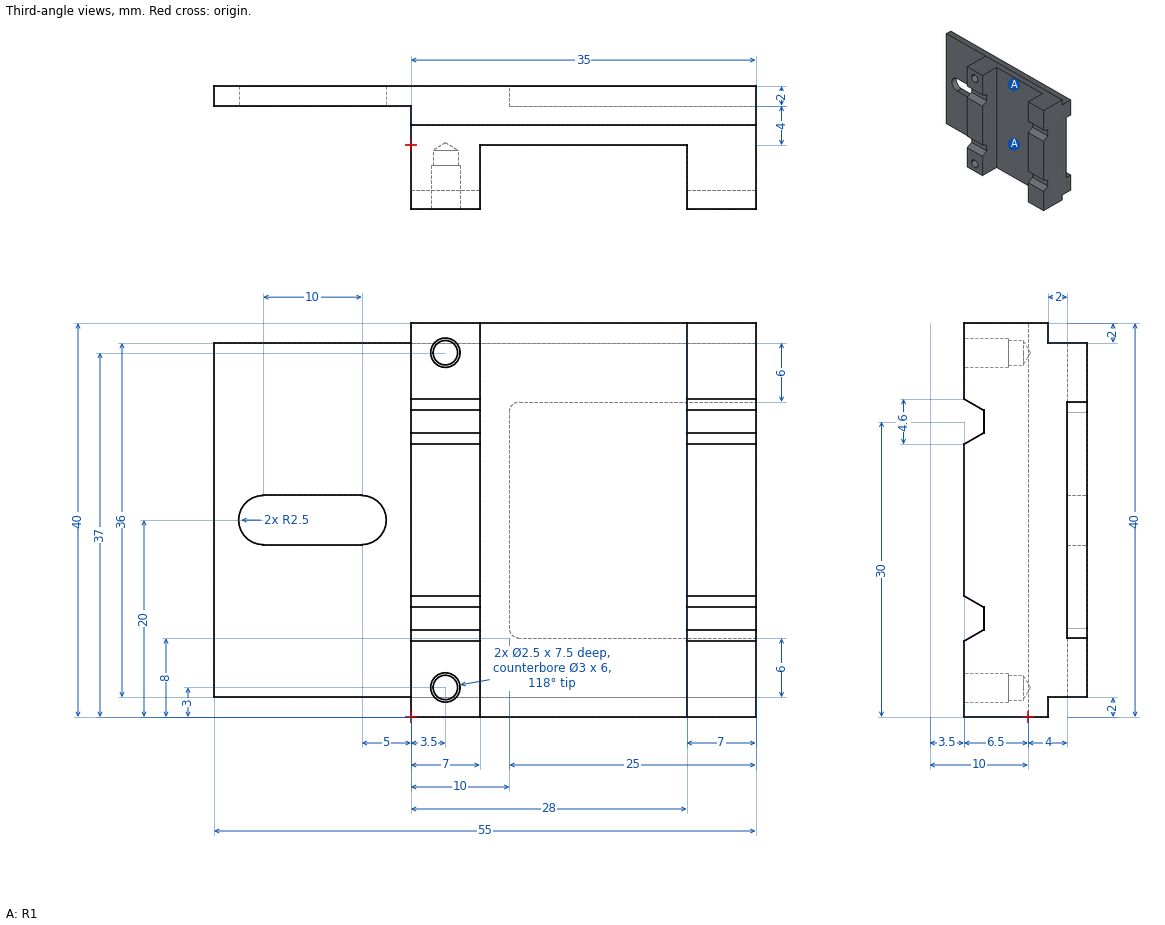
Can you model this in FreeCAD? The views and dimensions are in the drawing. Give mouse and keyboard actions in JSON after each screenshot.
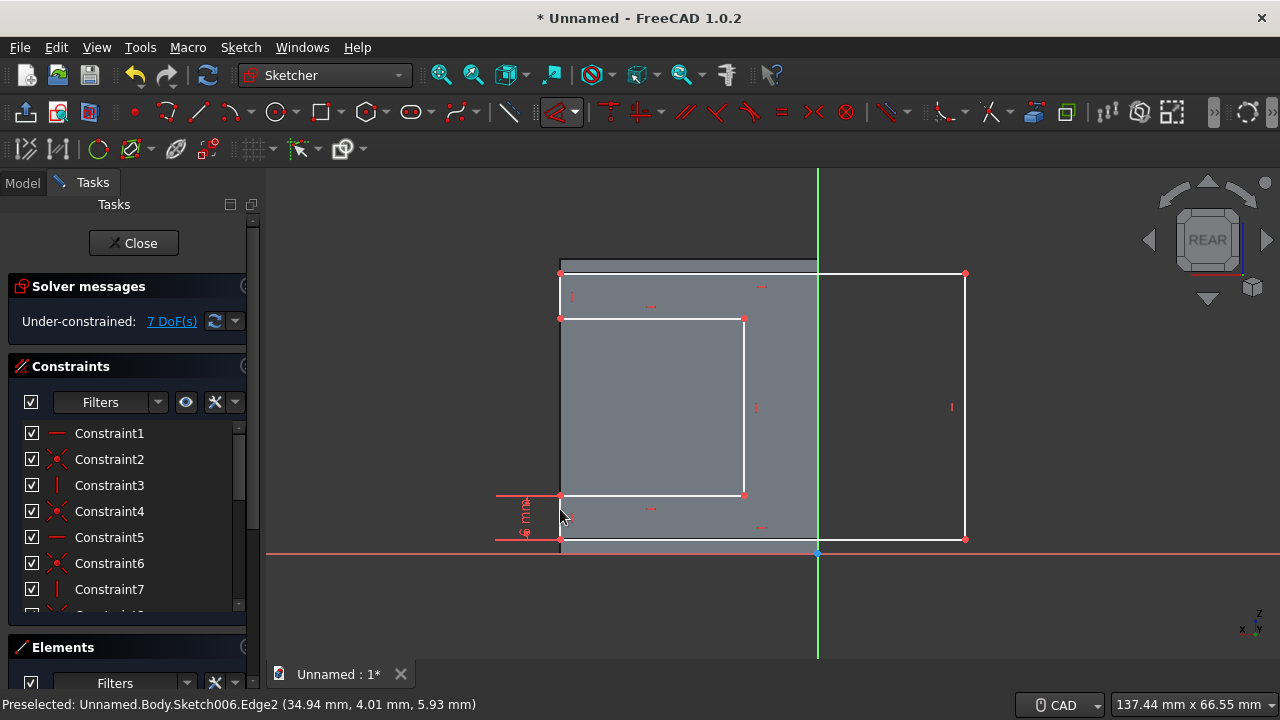
{"action": "left_click", "coordinate": [560, 288]}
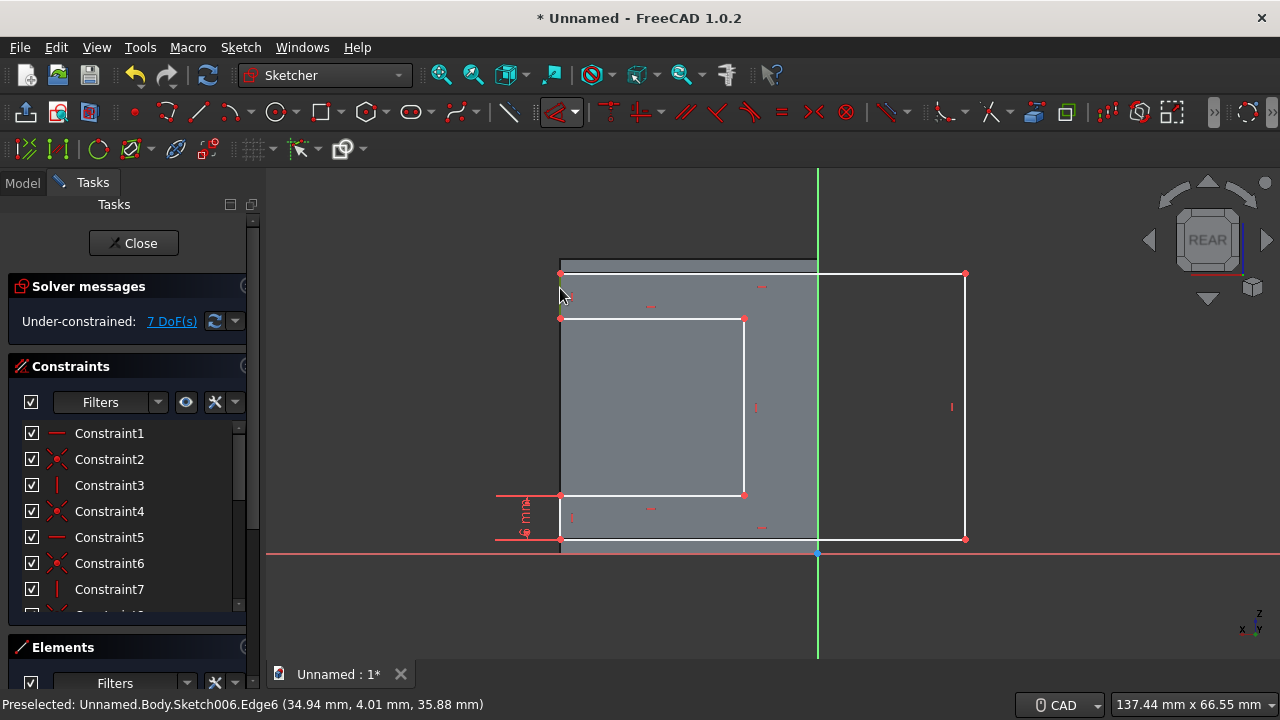
{"action": "left_click", "coordinate": [578, 112]}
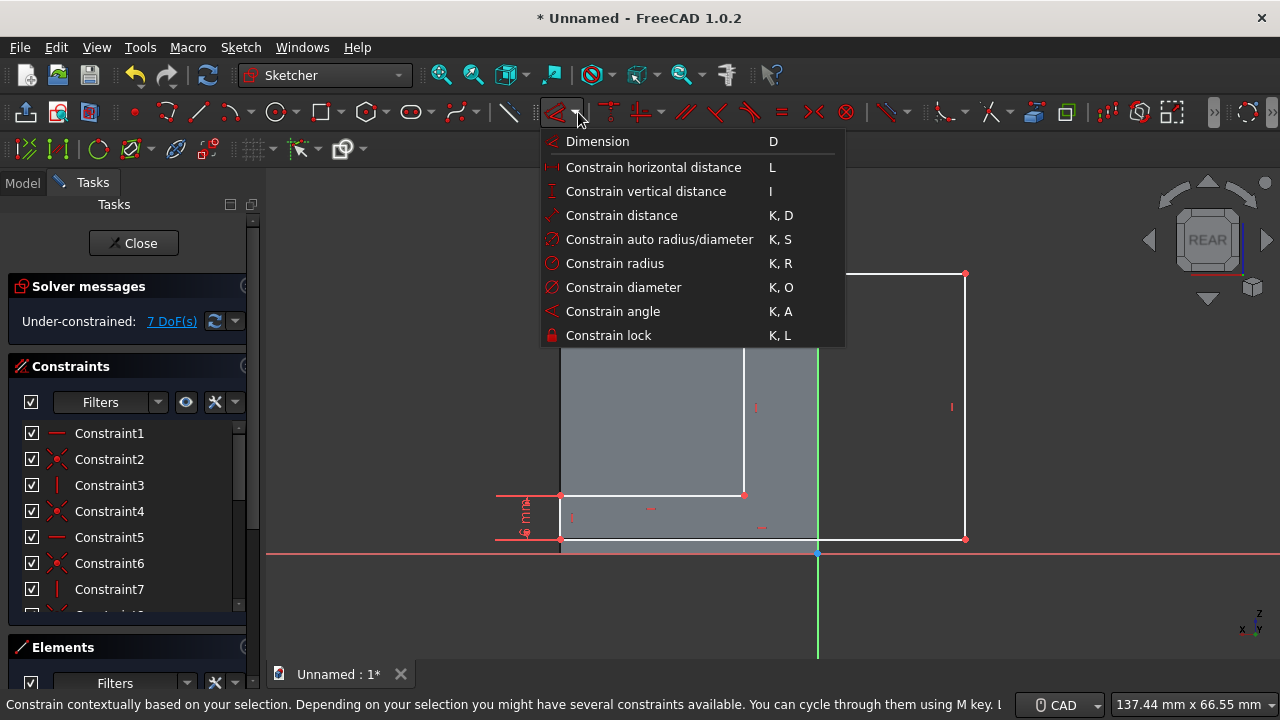
{"action": "left_click", "coordinate": [693, 191]}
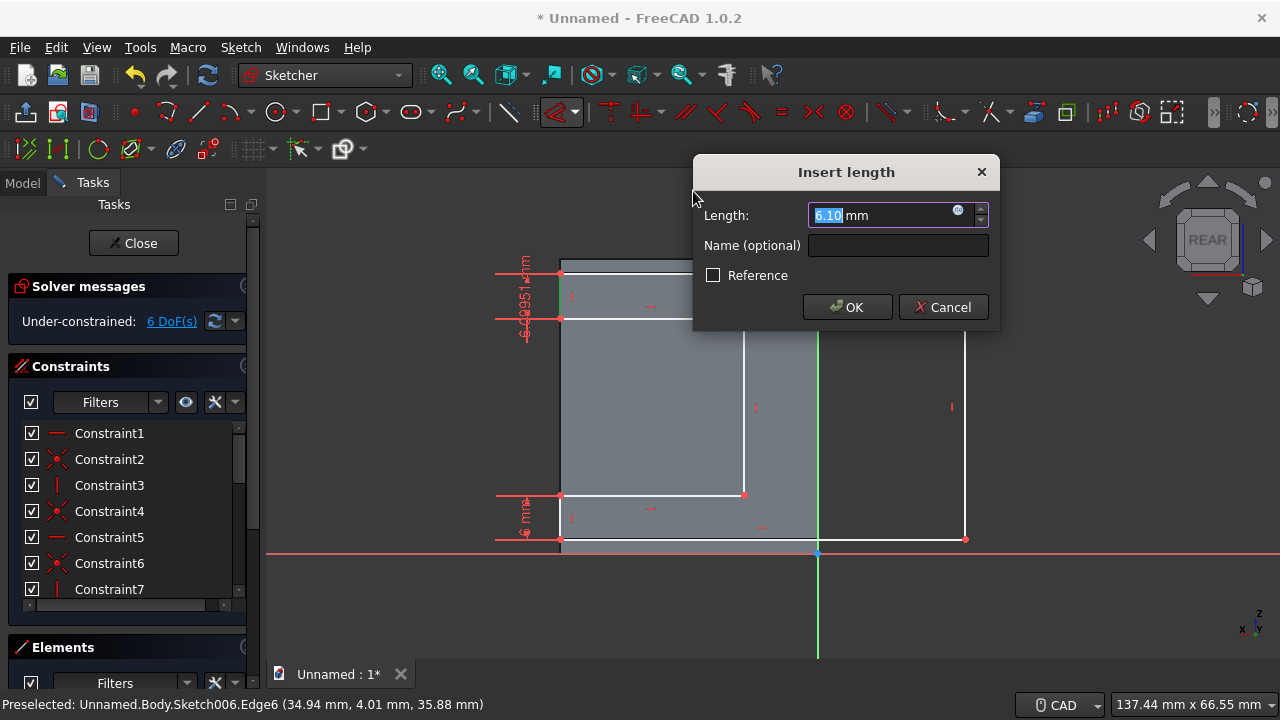
{"action": "type", "text": "6"}
{"action": "key", "text": "Return"}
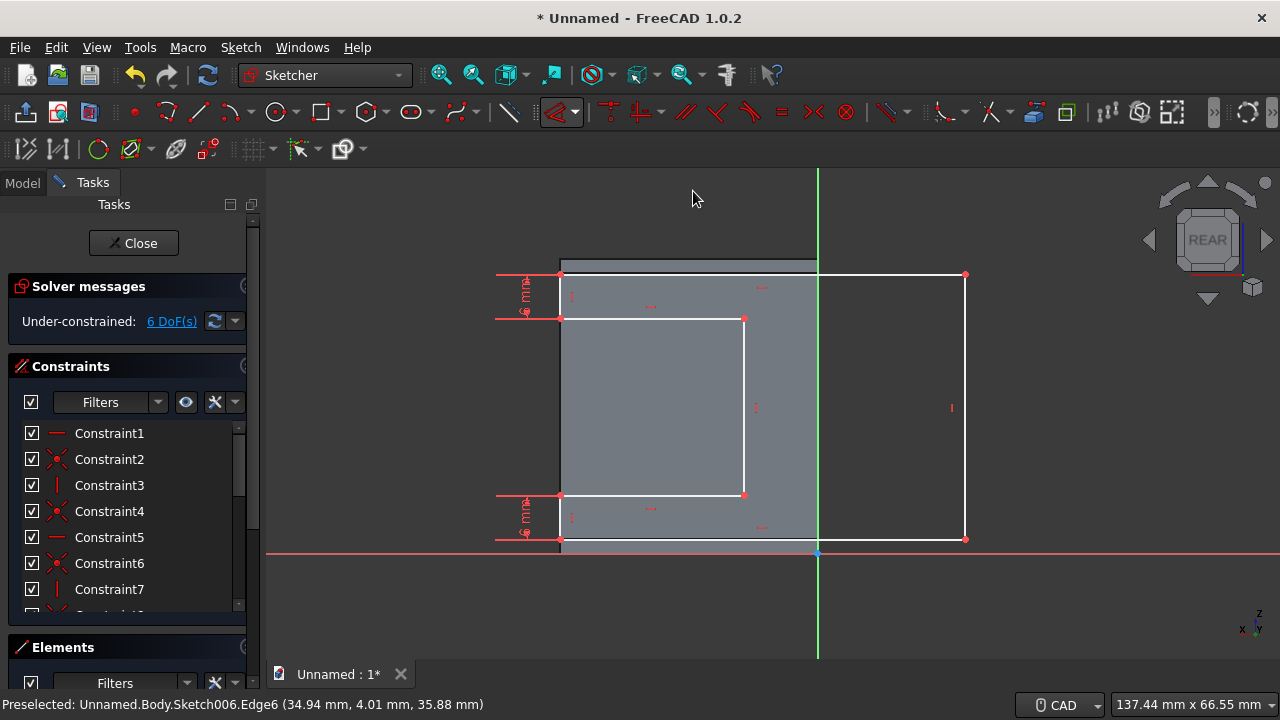
{"action": "left_click", "coordinate": [689, 496]}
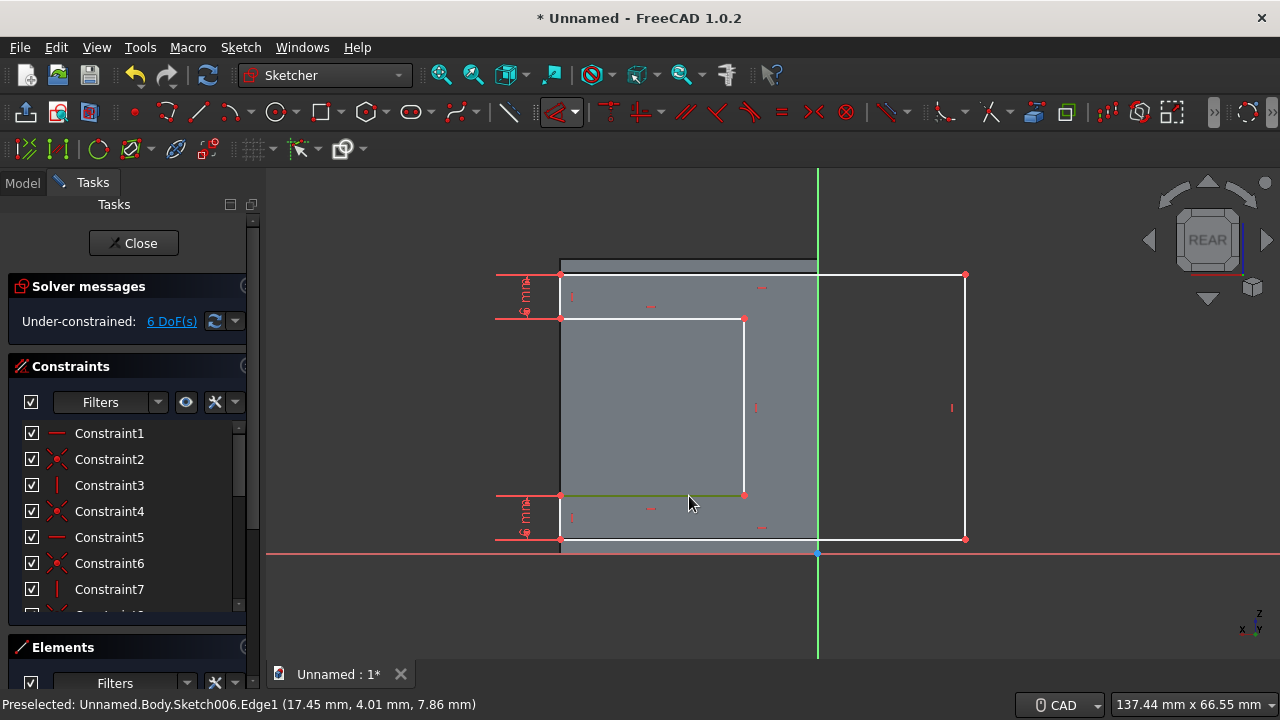
{"action": "key", "text": "l"}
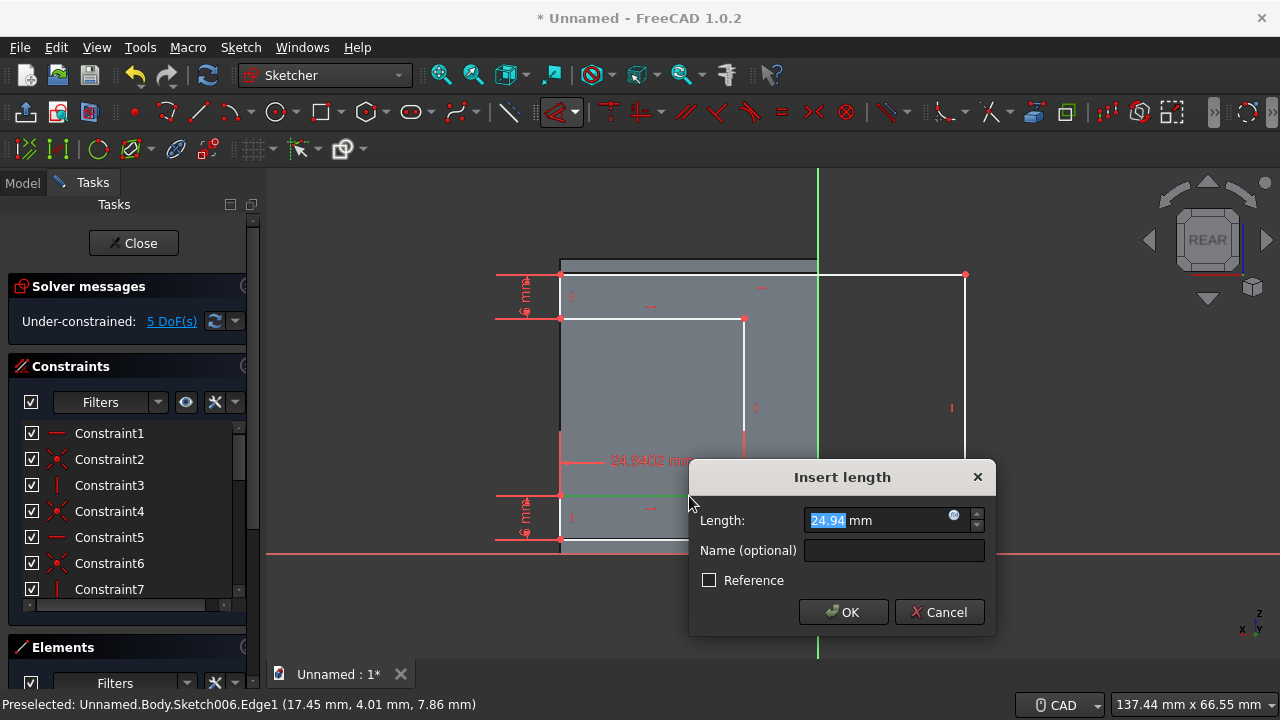
{"action": "type", "text": "25"}
{"action": "key", "text": "Return"}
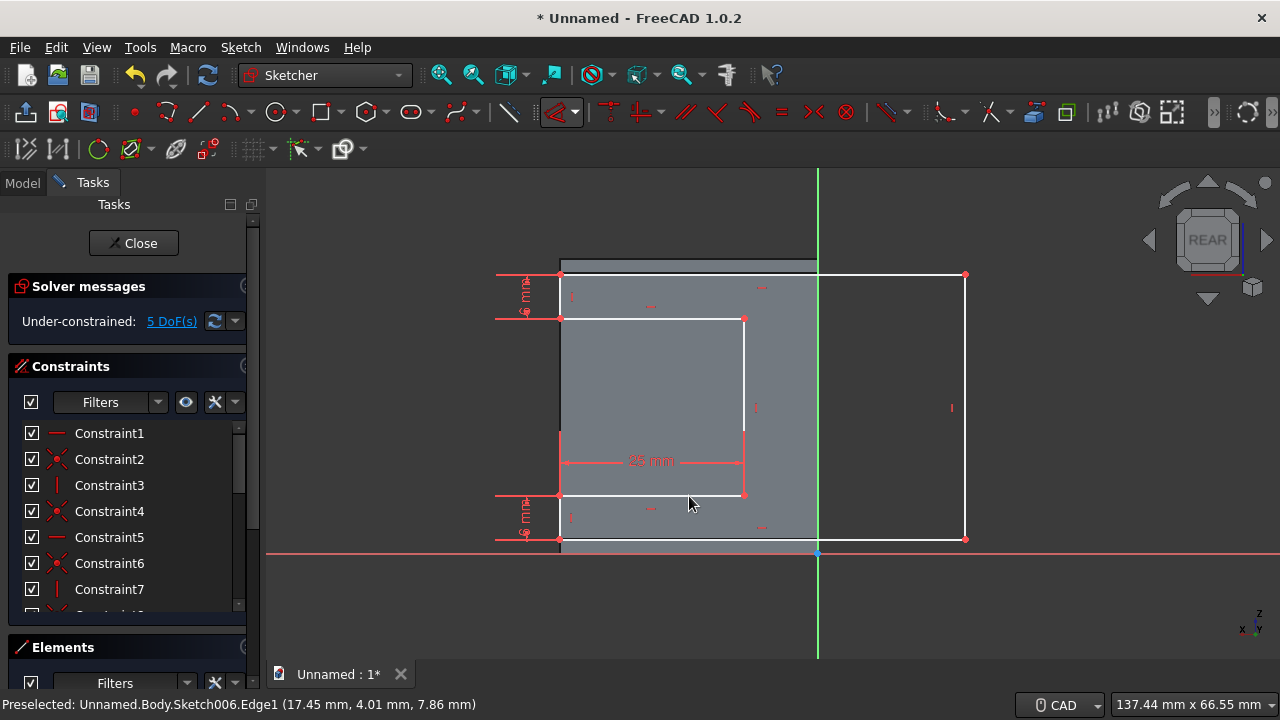
{"action": "left_click", "coordinate": [681, 540]}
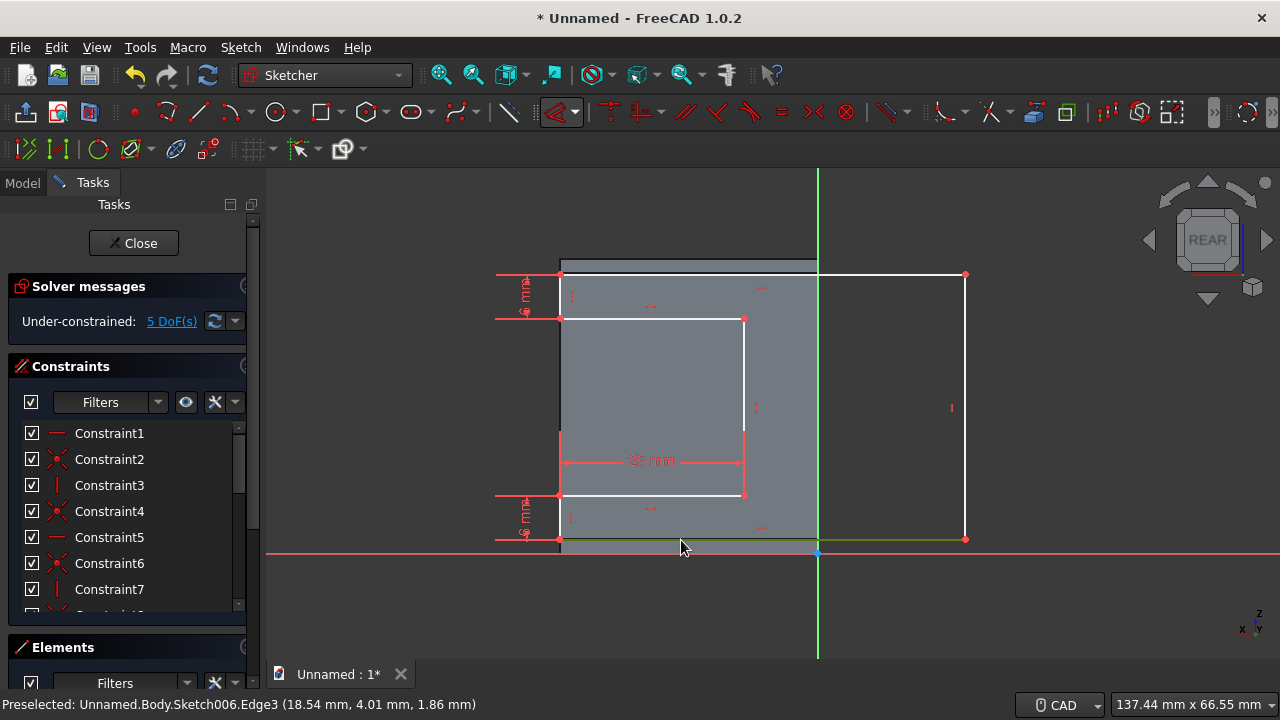
{"action": "left_click", "coordinate": [578, 112]}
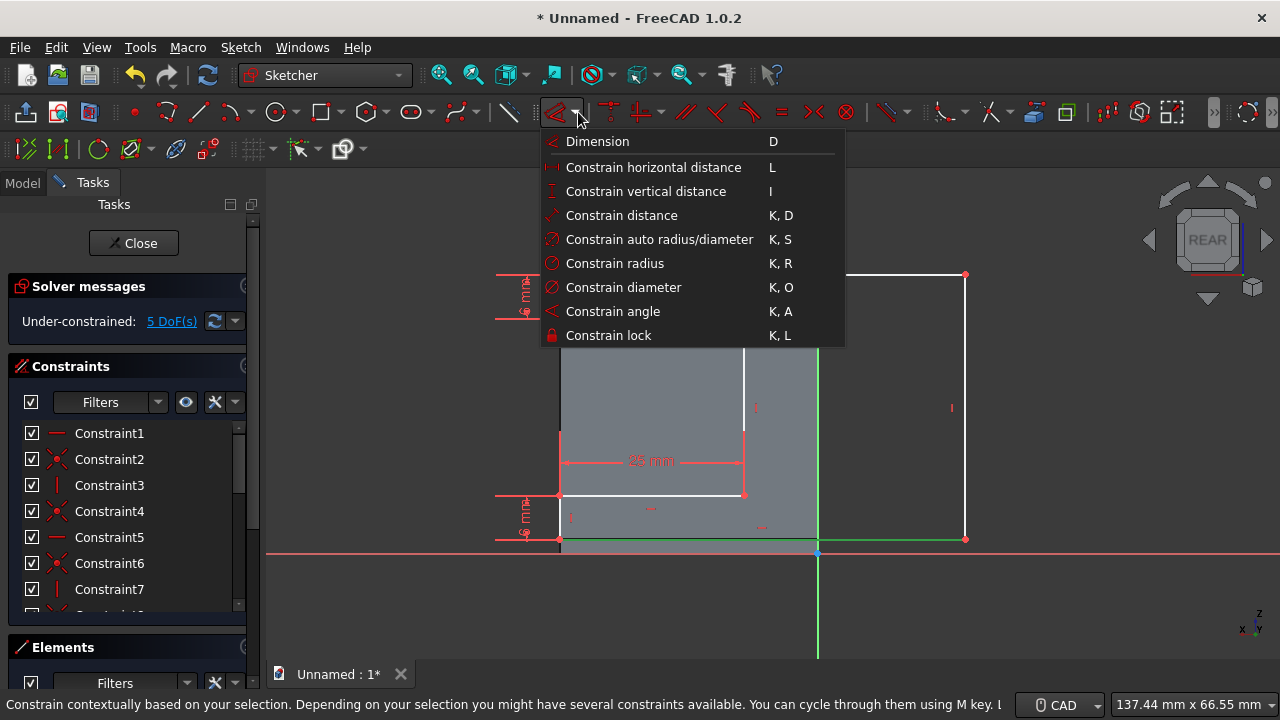
{"action": "left_click", "coordinate": [693, 167]}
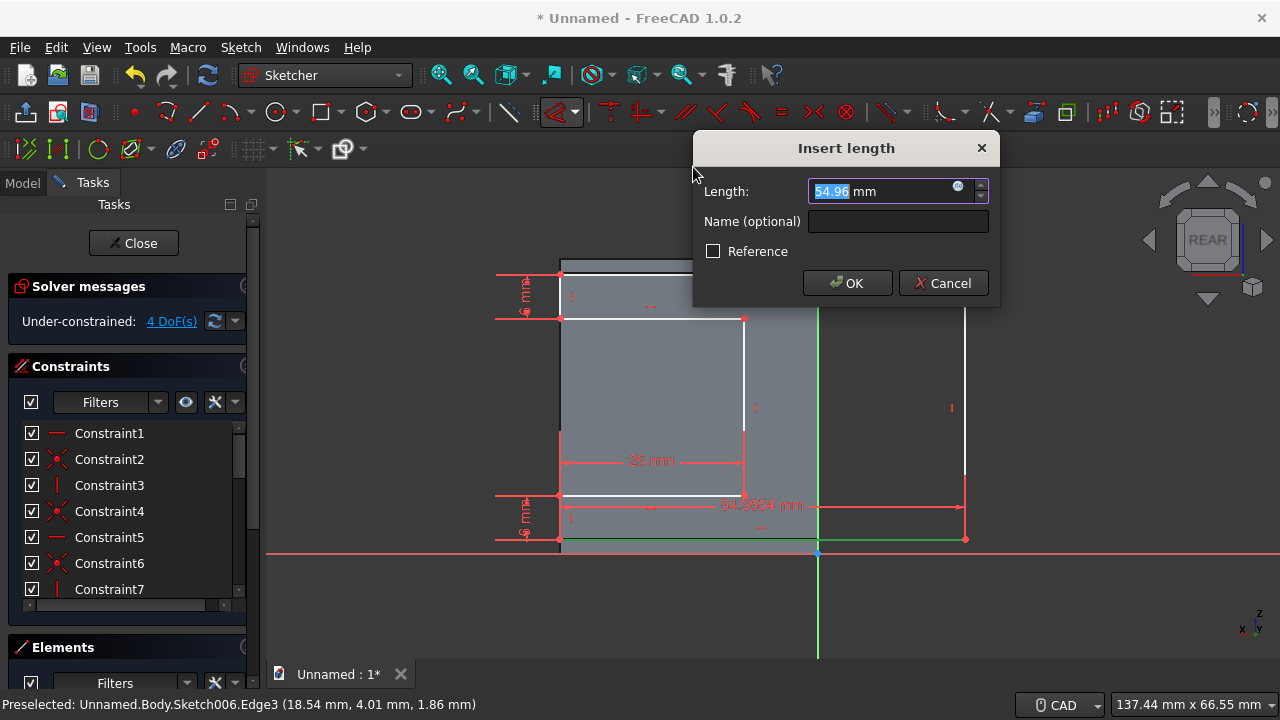
{"action": "type", "text": "55"}
{"action": "key", "text": "Return"}